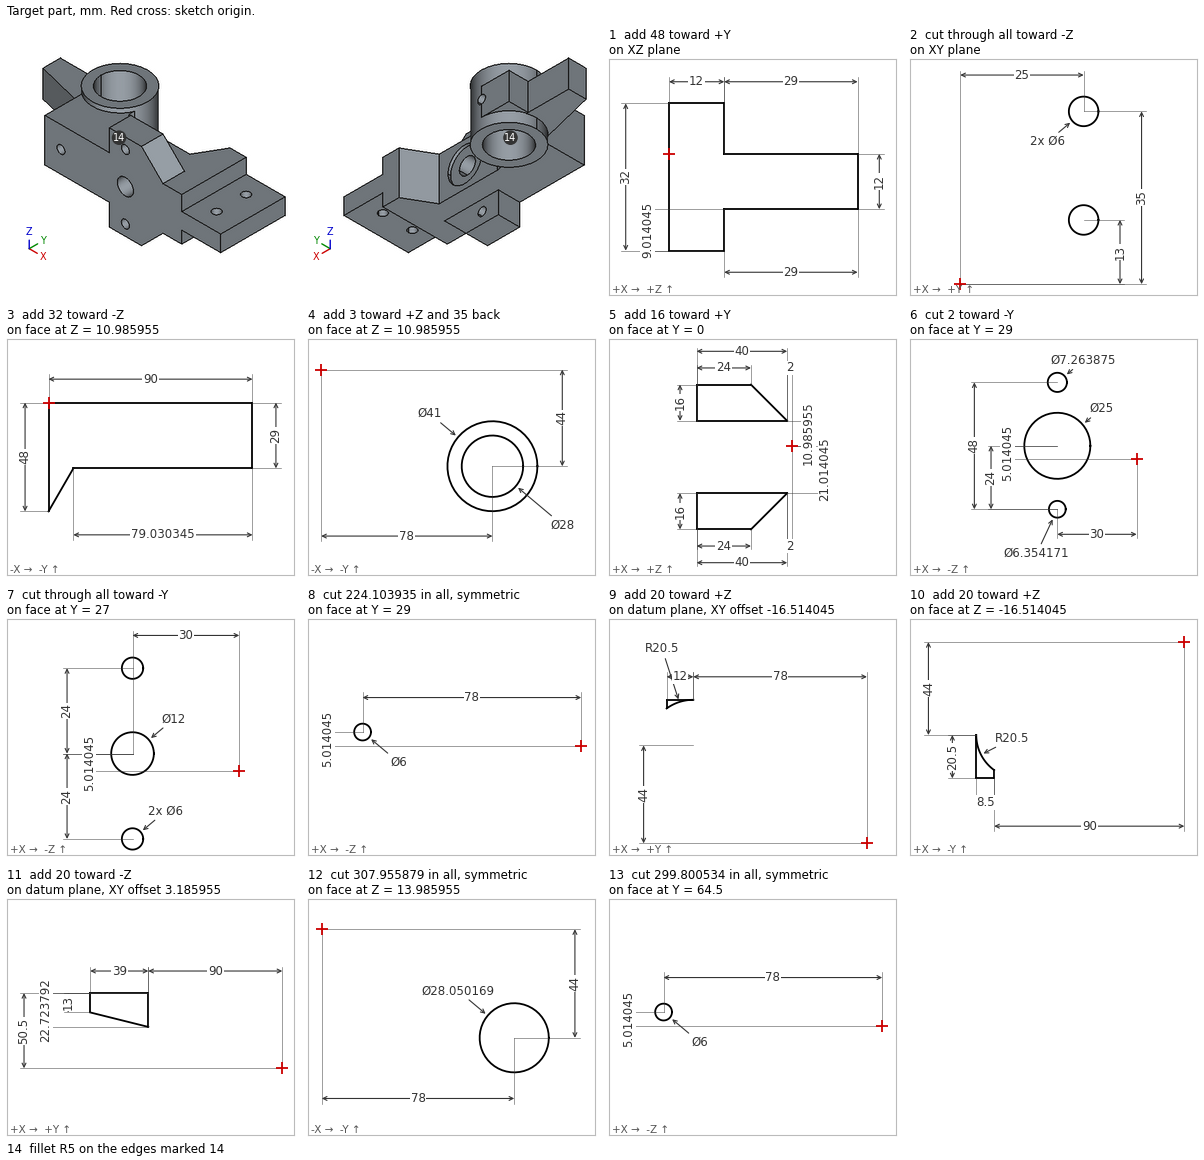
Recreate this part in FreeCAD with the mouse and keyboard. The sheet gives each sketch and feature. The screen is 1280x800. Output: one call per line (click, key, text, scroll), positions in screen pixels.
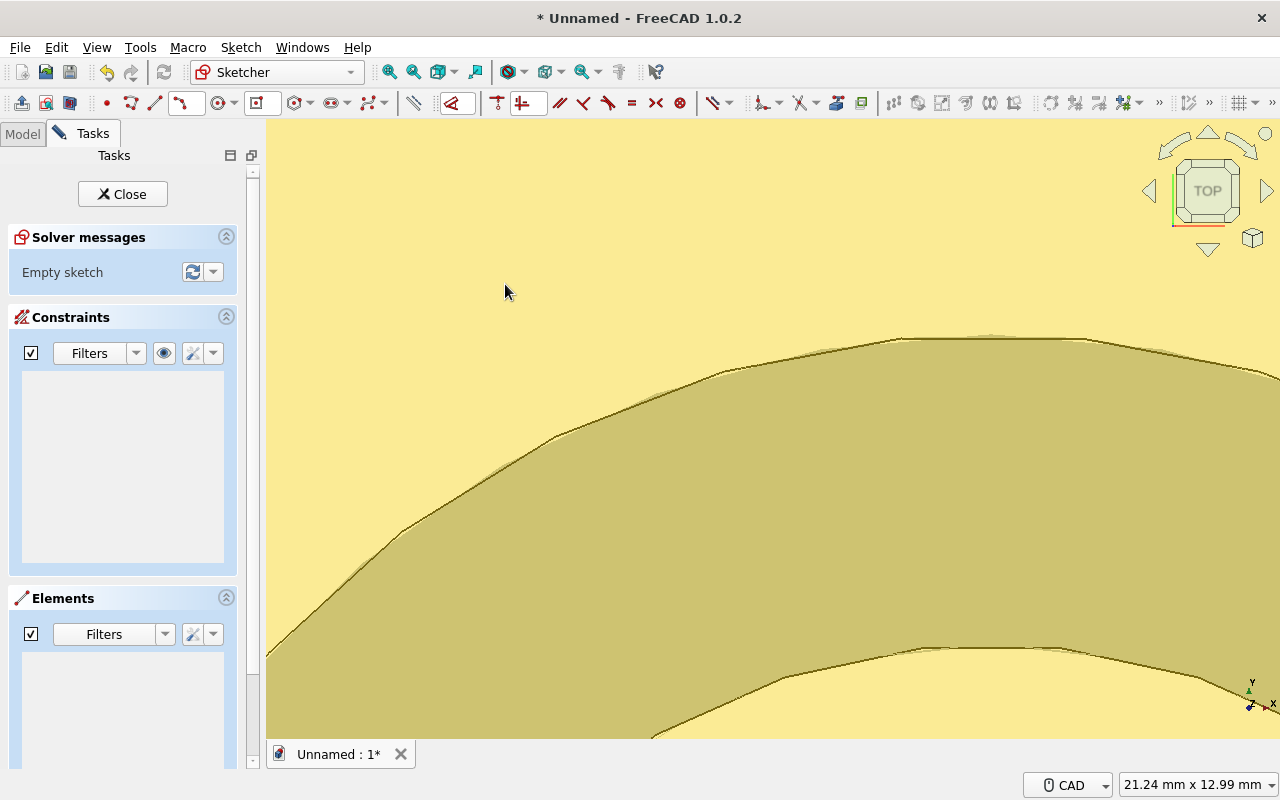
key(g)
key(m)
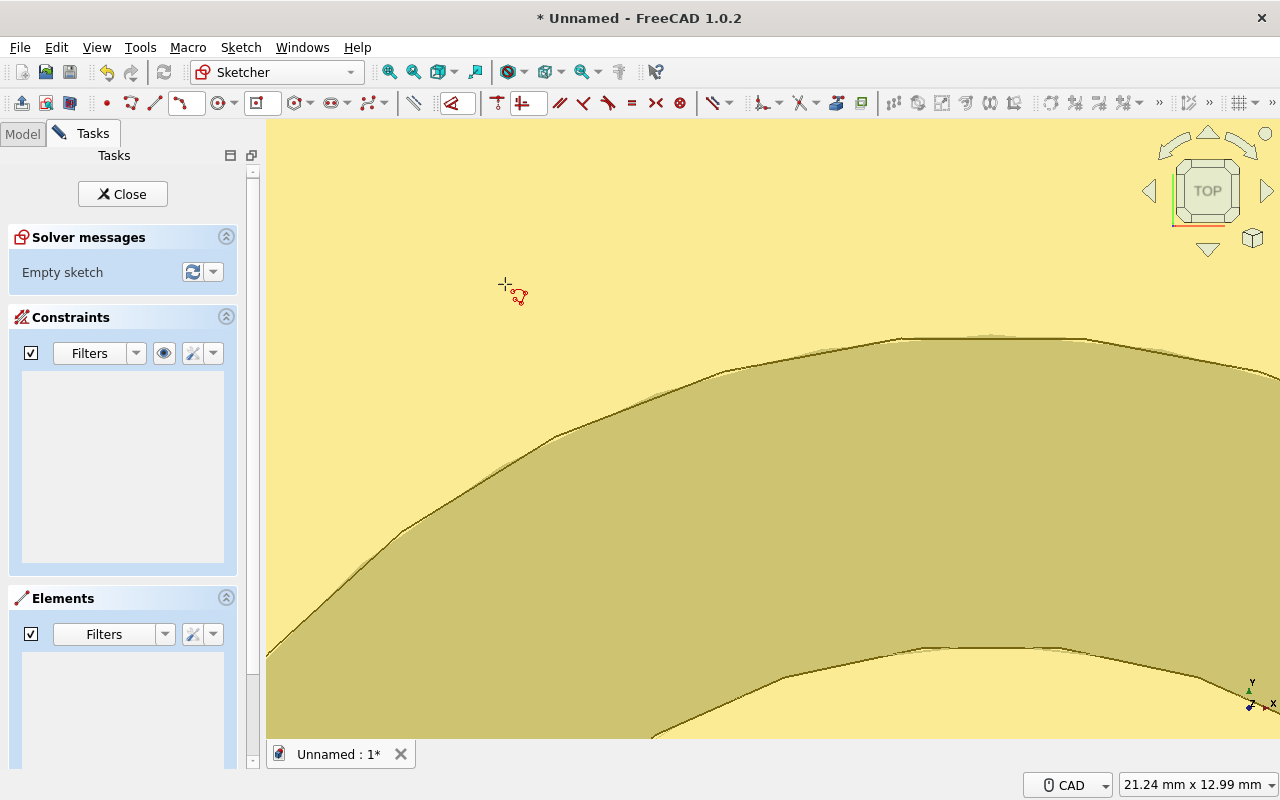
click(991, 334)
click(419, 334)
click(419, 520)
right_click(419, 520)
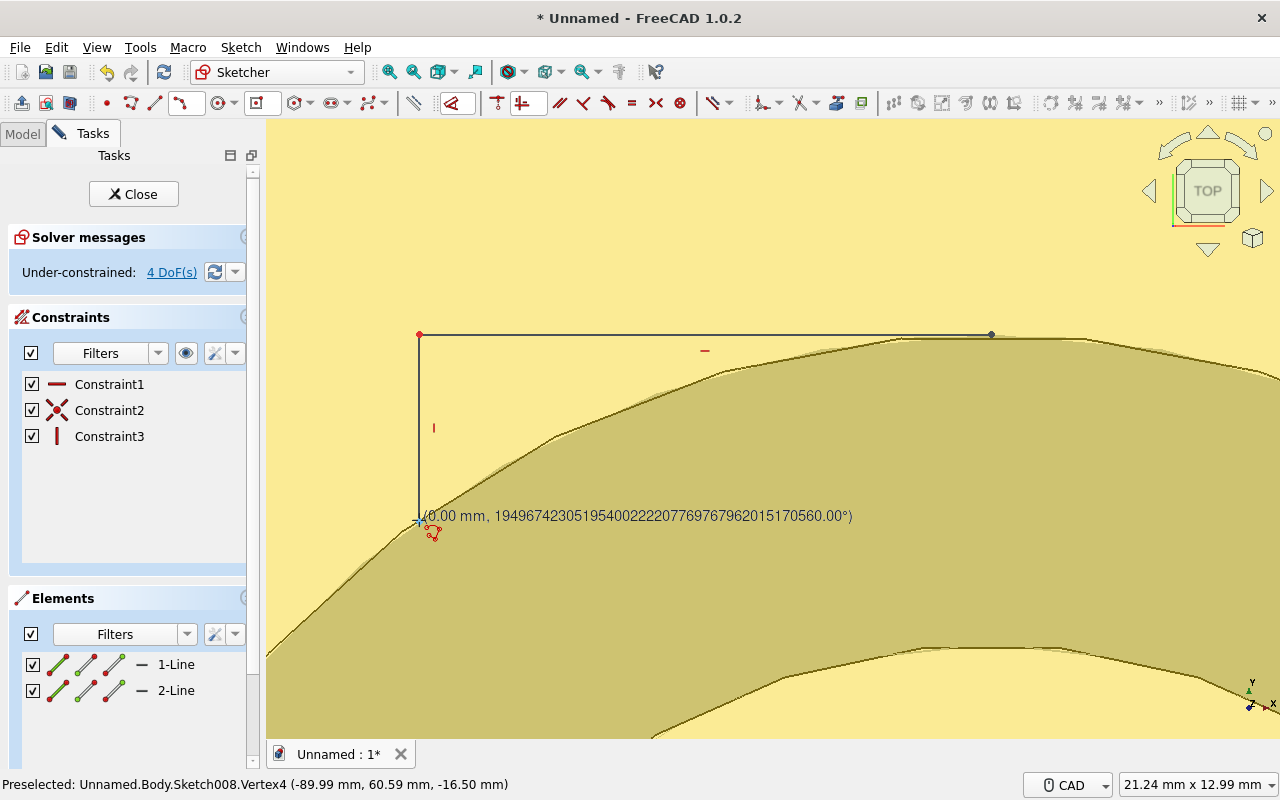
click(180, 104)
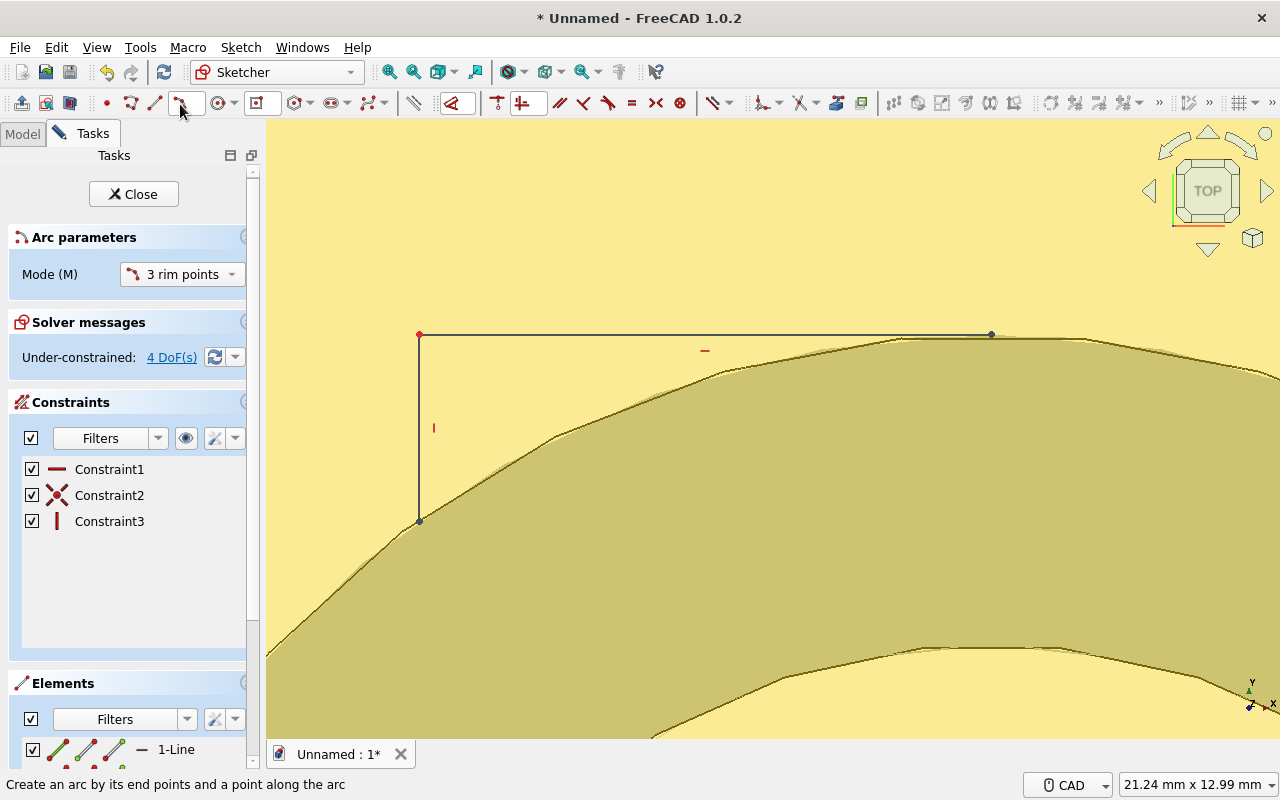
click(419, 521)
click(991, 335)
click(690, 382)
key(Escape)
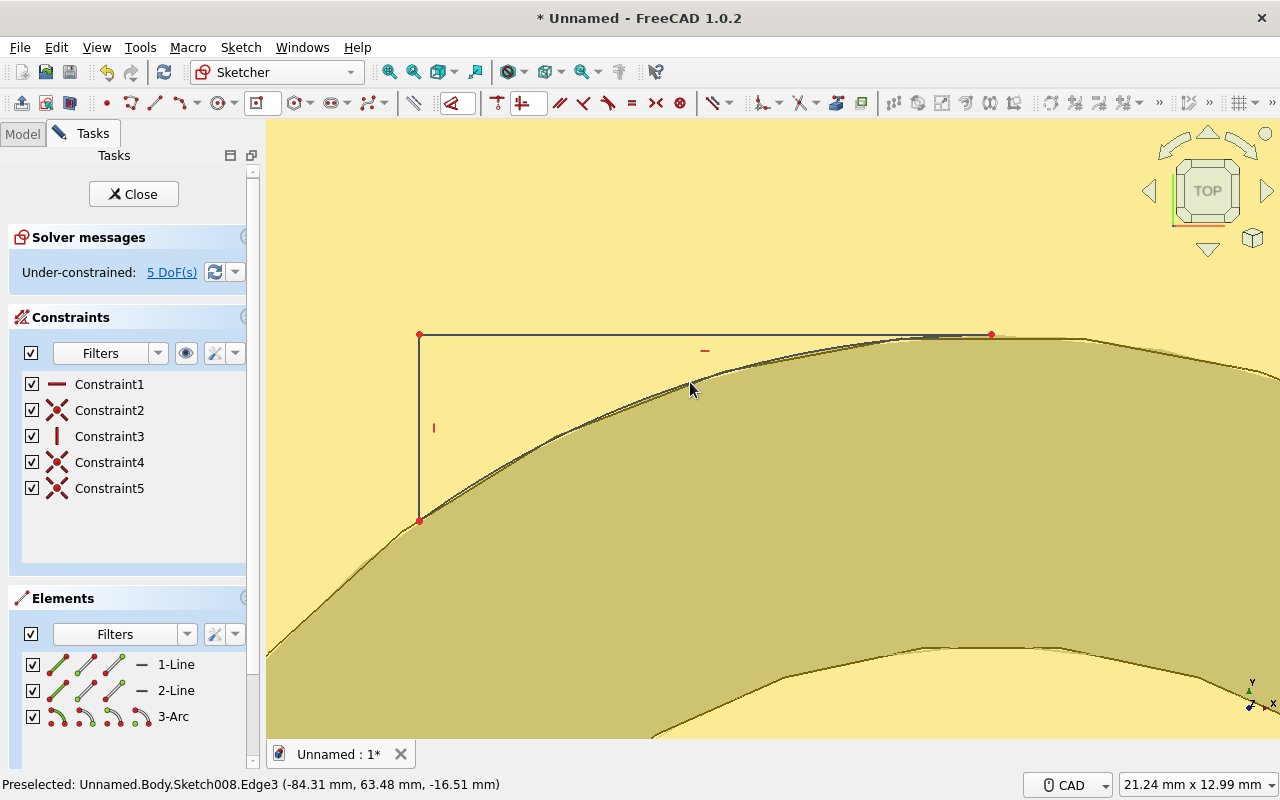
click(819, 335)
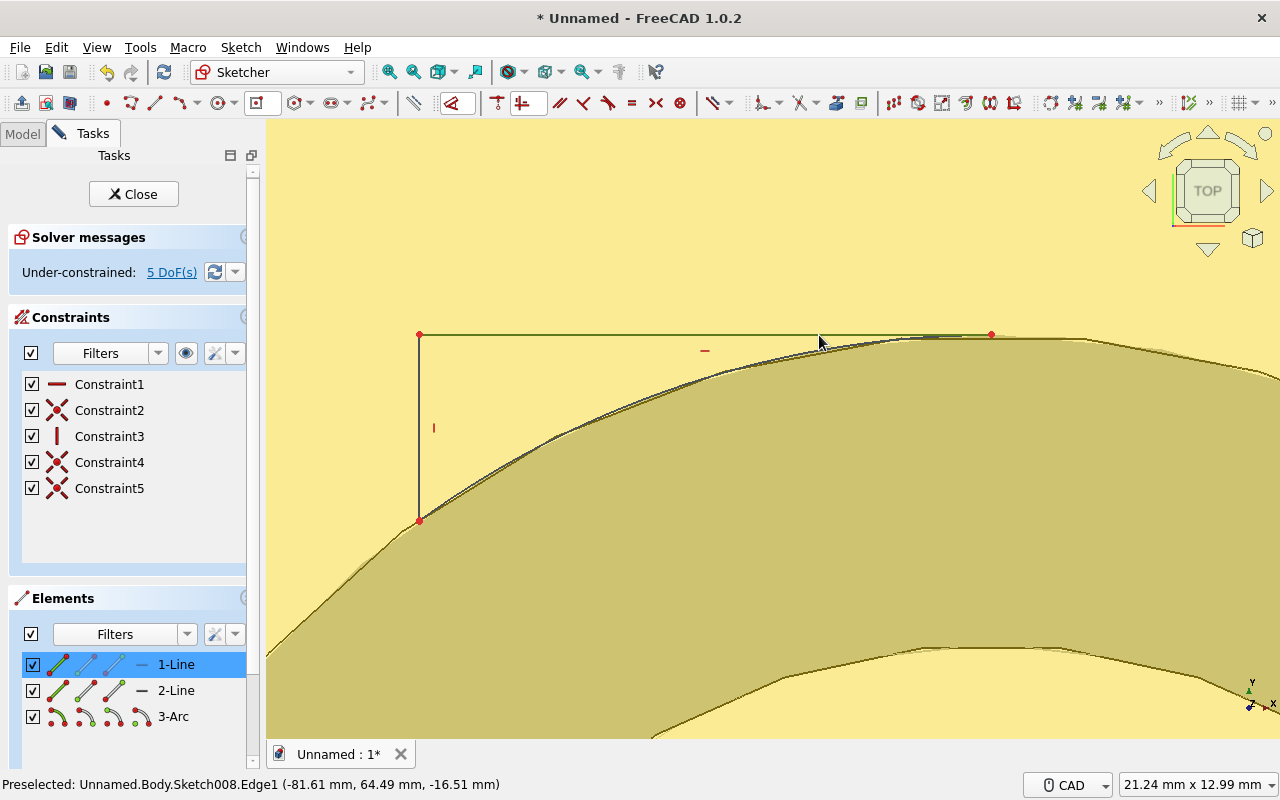
click(809, 352)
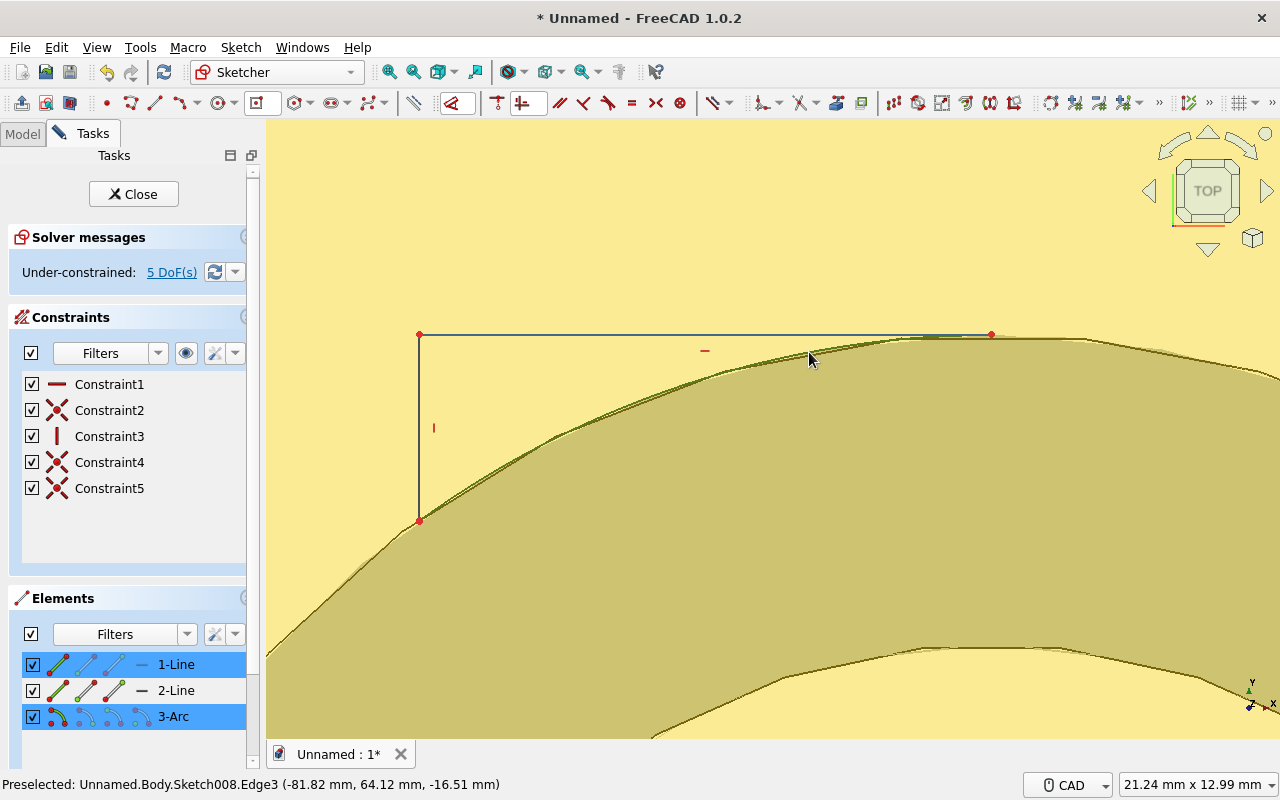
key(t)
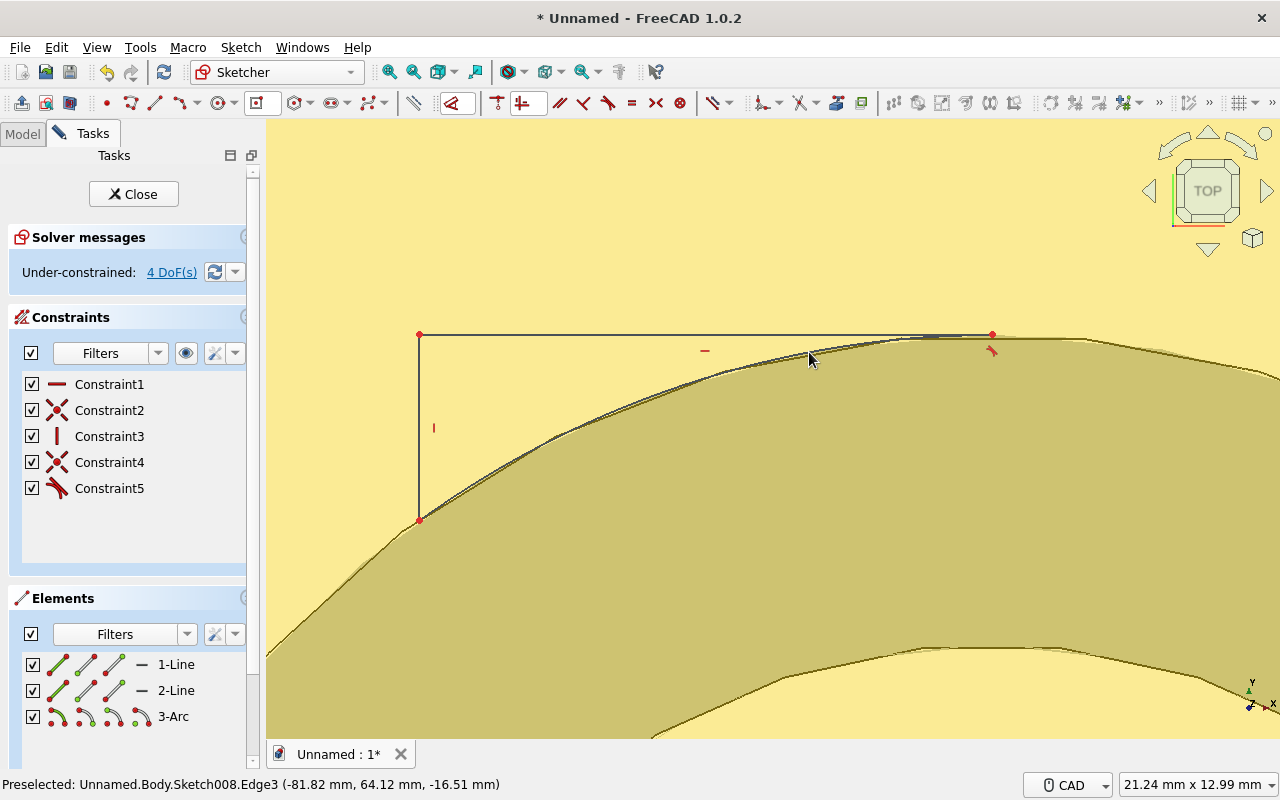
click(810, 352)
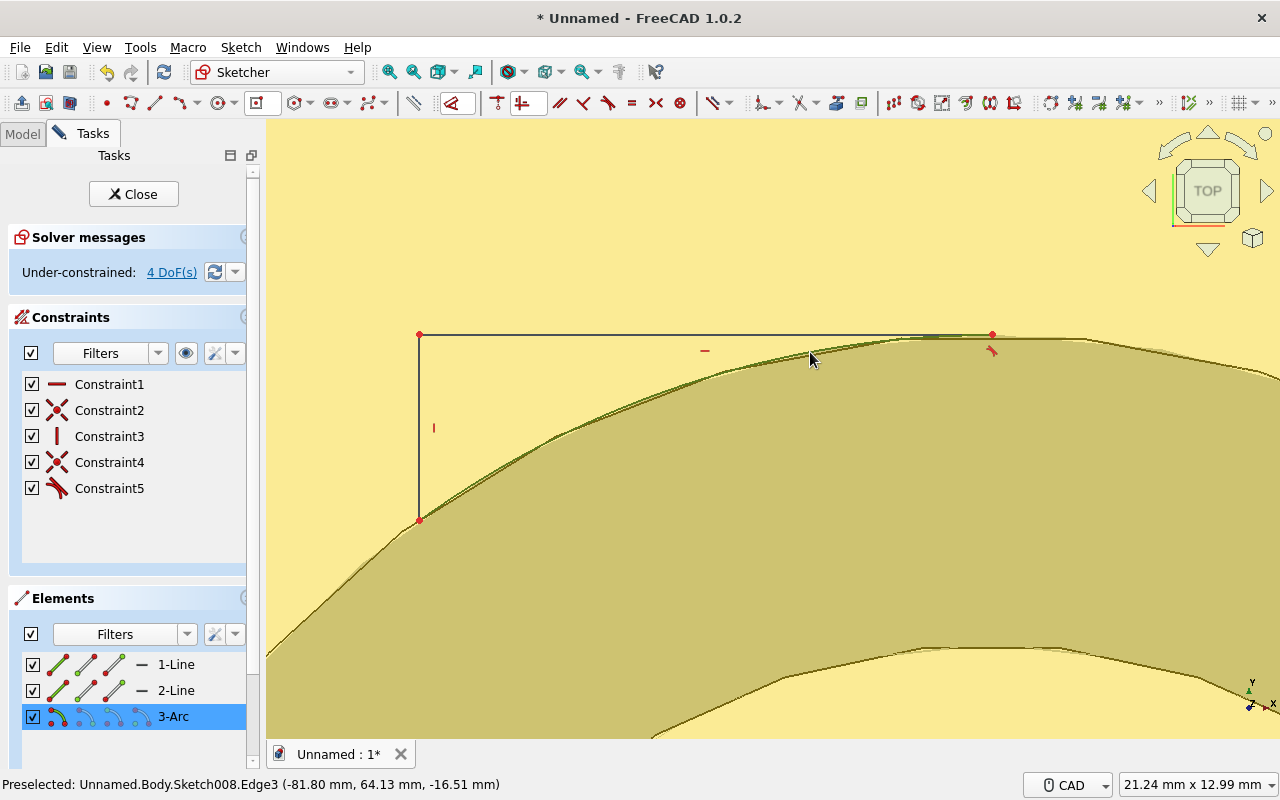
click(470, 104)